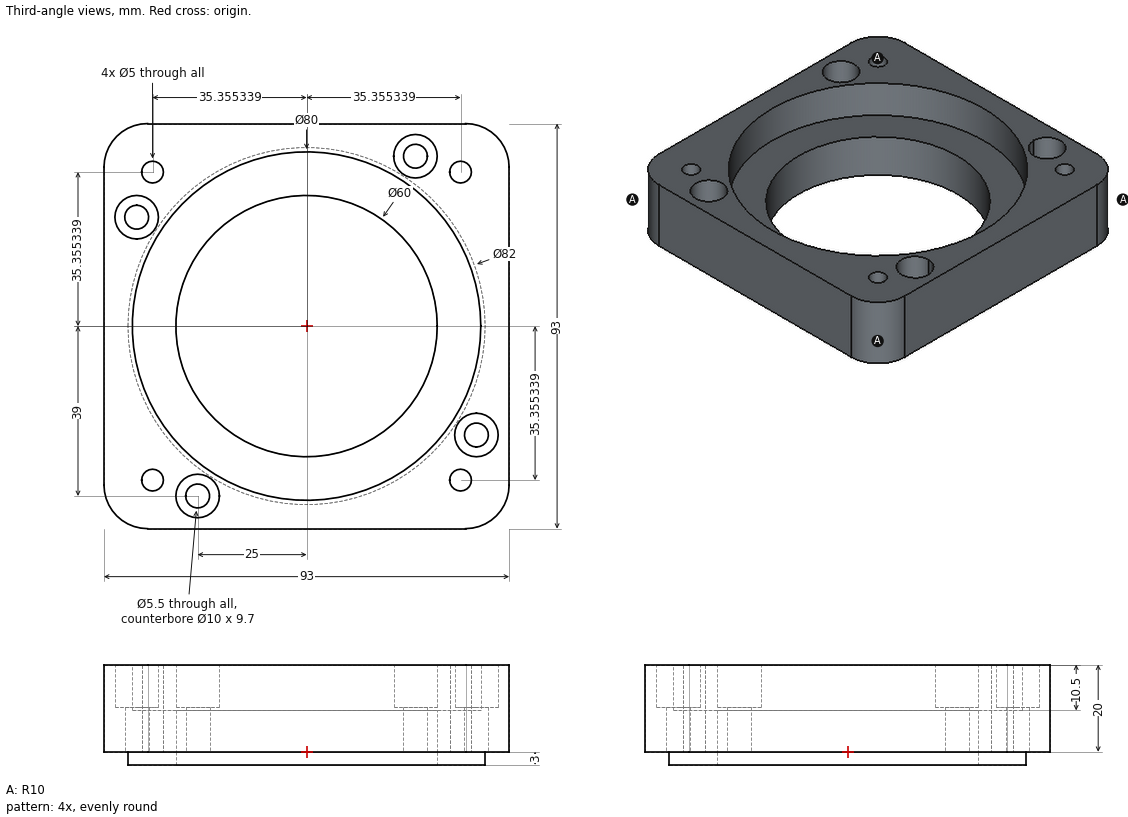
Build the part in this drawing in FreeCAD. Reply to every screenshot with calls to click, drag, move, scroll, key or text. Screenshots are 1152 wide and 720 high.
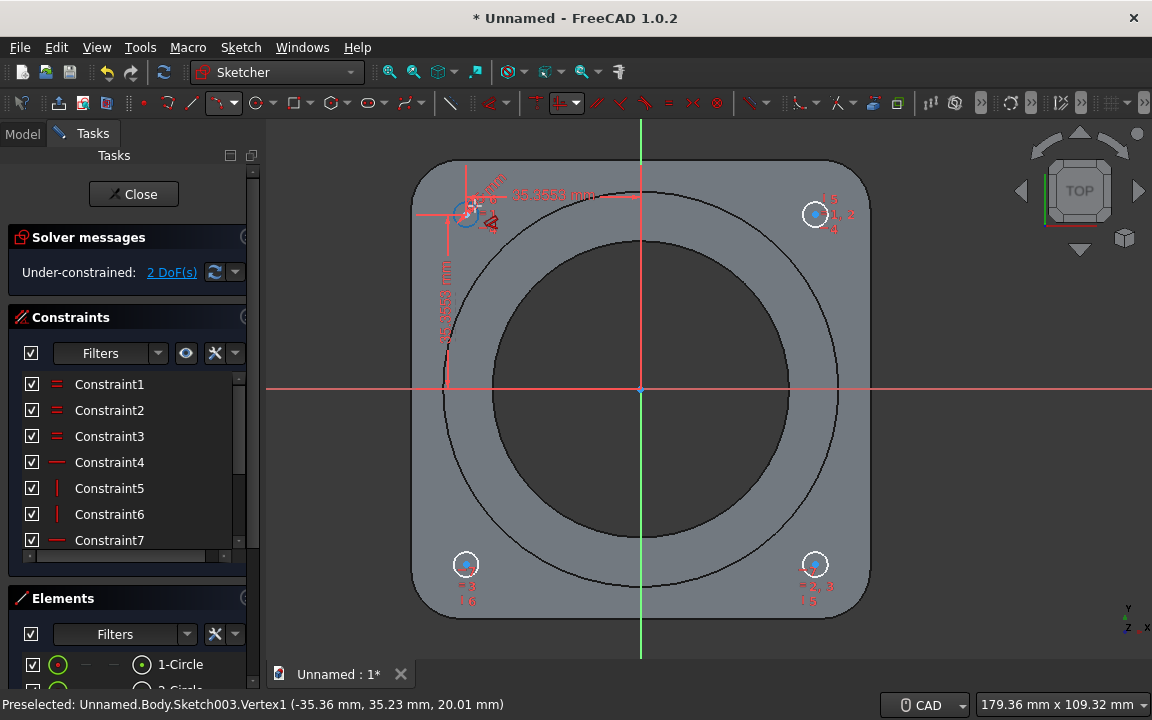
click(815, 215)
click(728, 181)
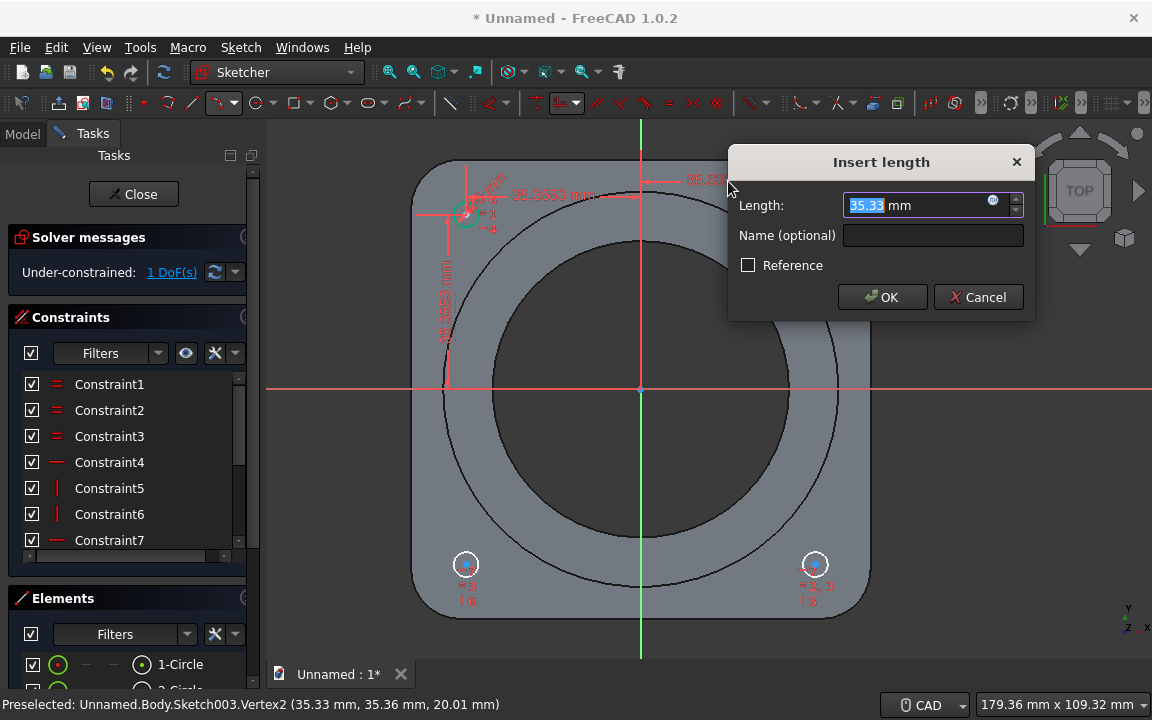
text(35.355339)
key(Return)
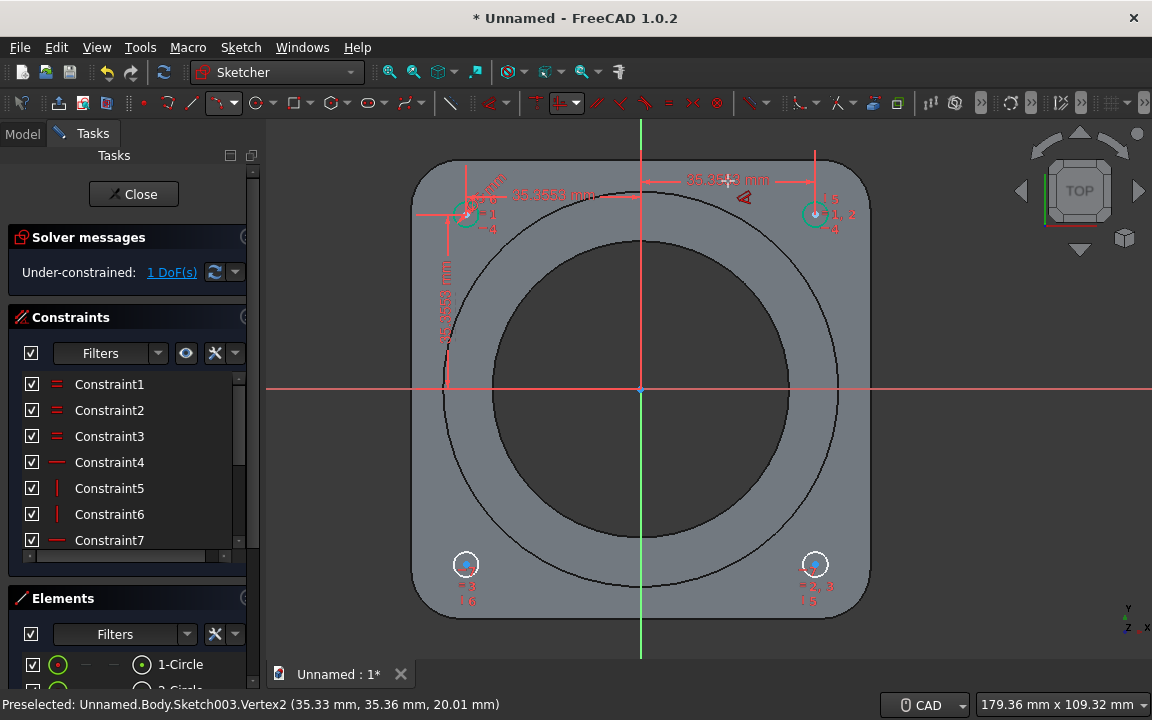
click(815, 565)
click(849, 477)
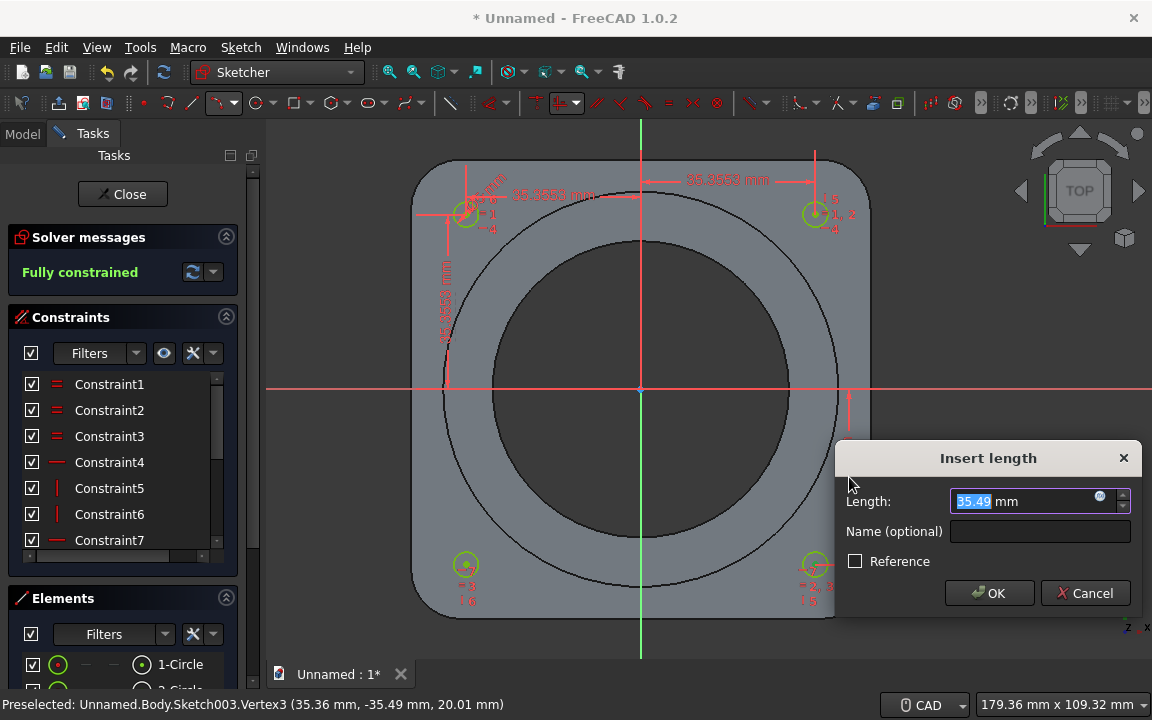
text(35.355339)
key(Return)
key(Escape)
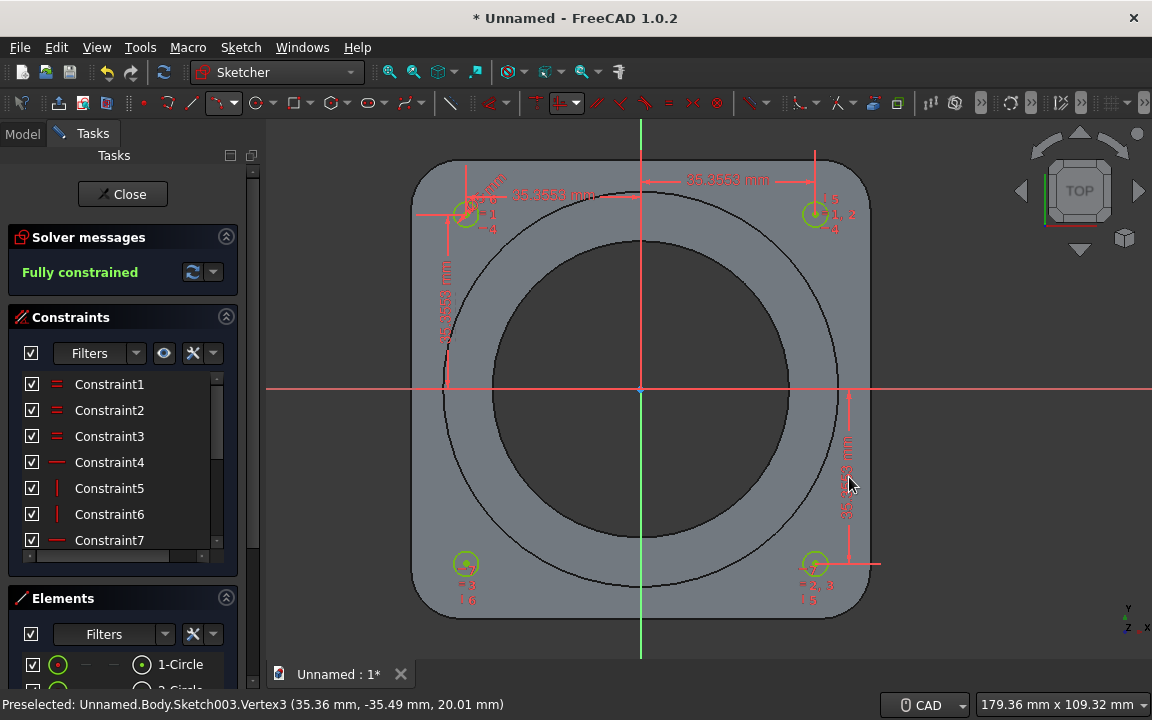
click(123, 194)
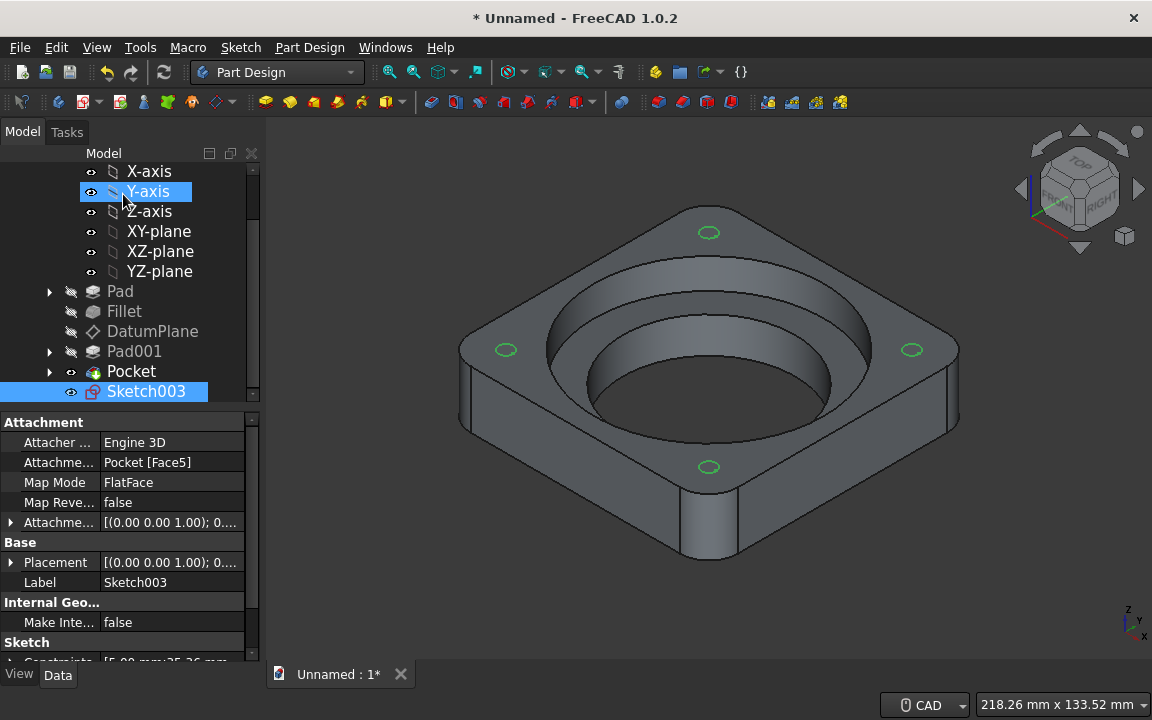
click(456, 102)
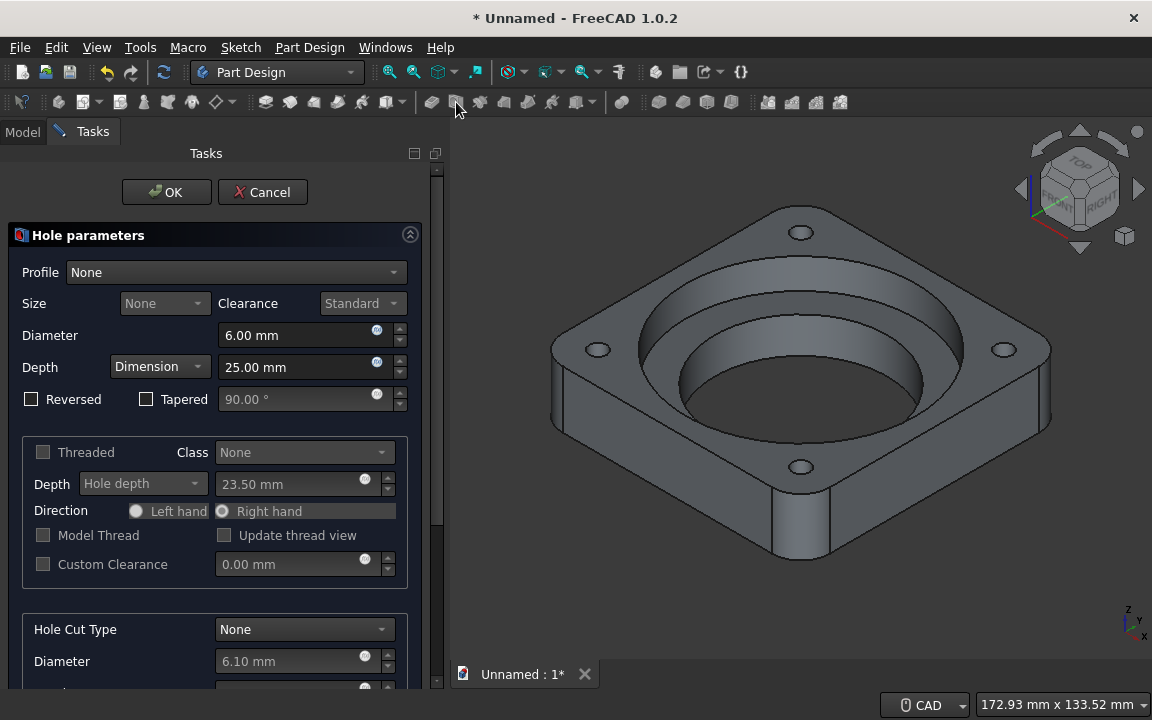
triple_click(305, 335)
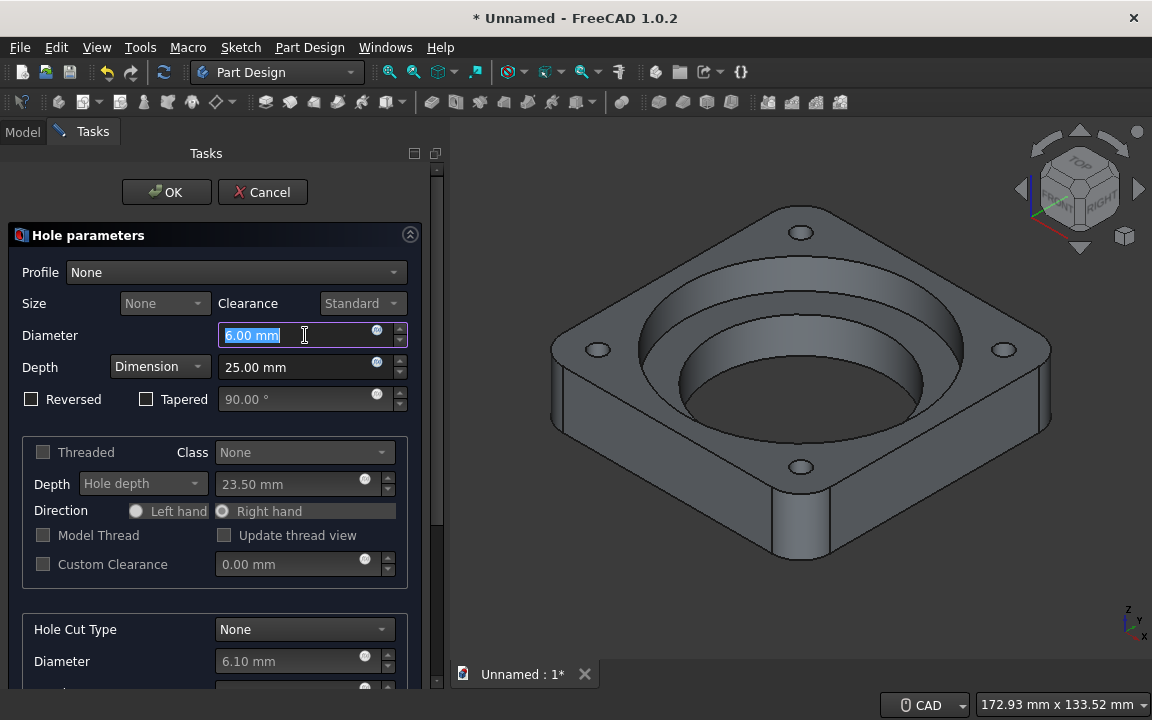
text(5)
key(Tab)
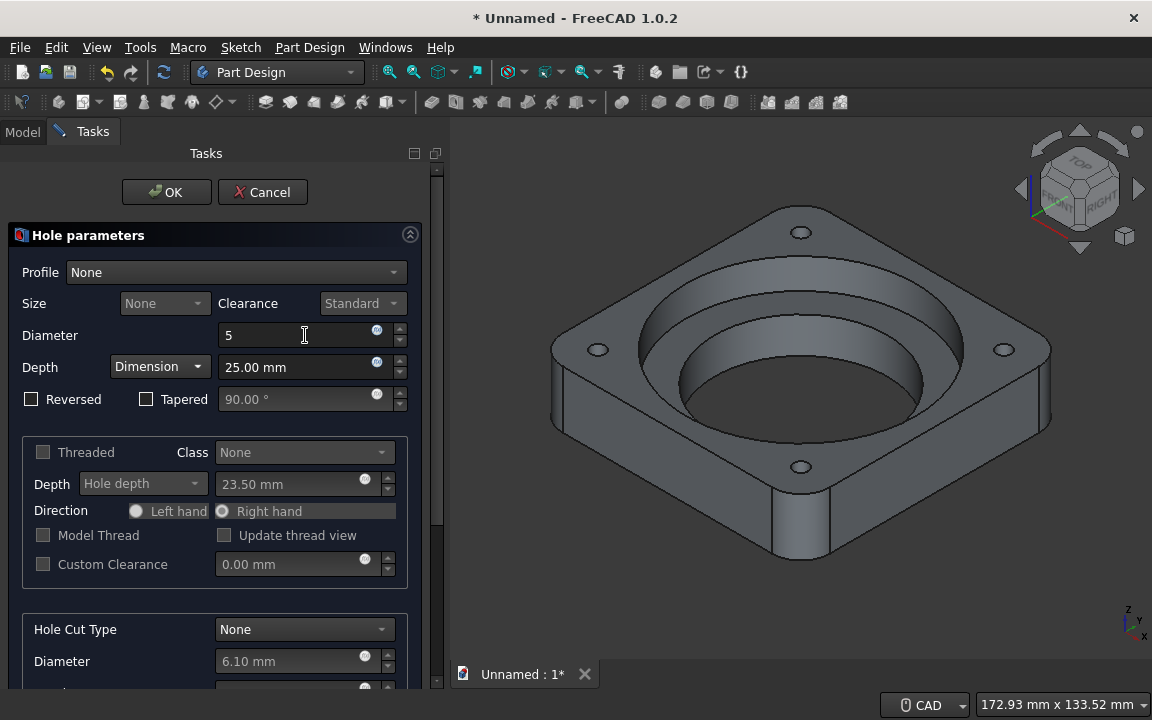
click(161, 366)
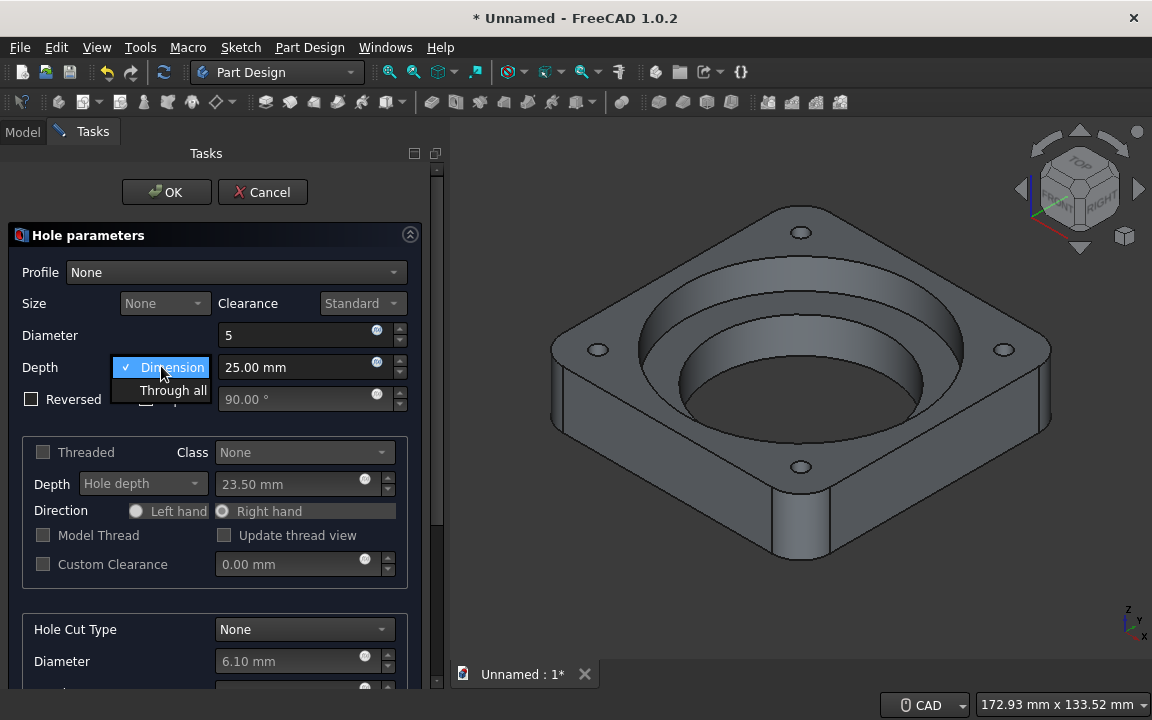
click(160, 390)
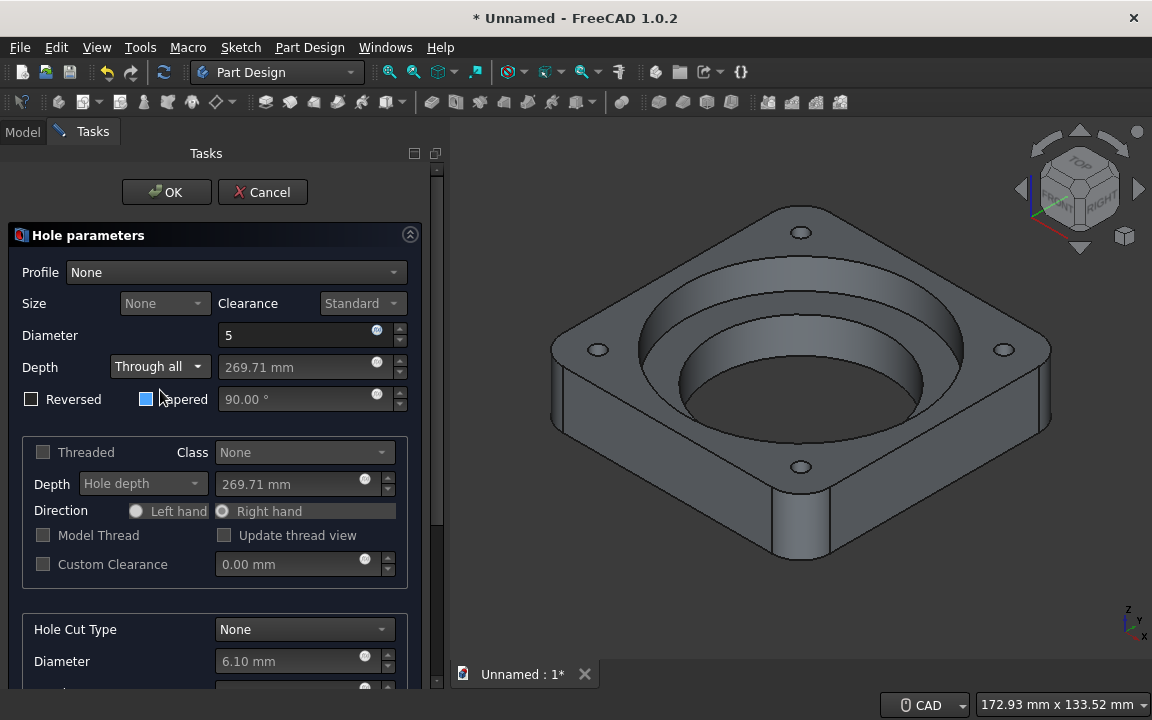
click(167, 192)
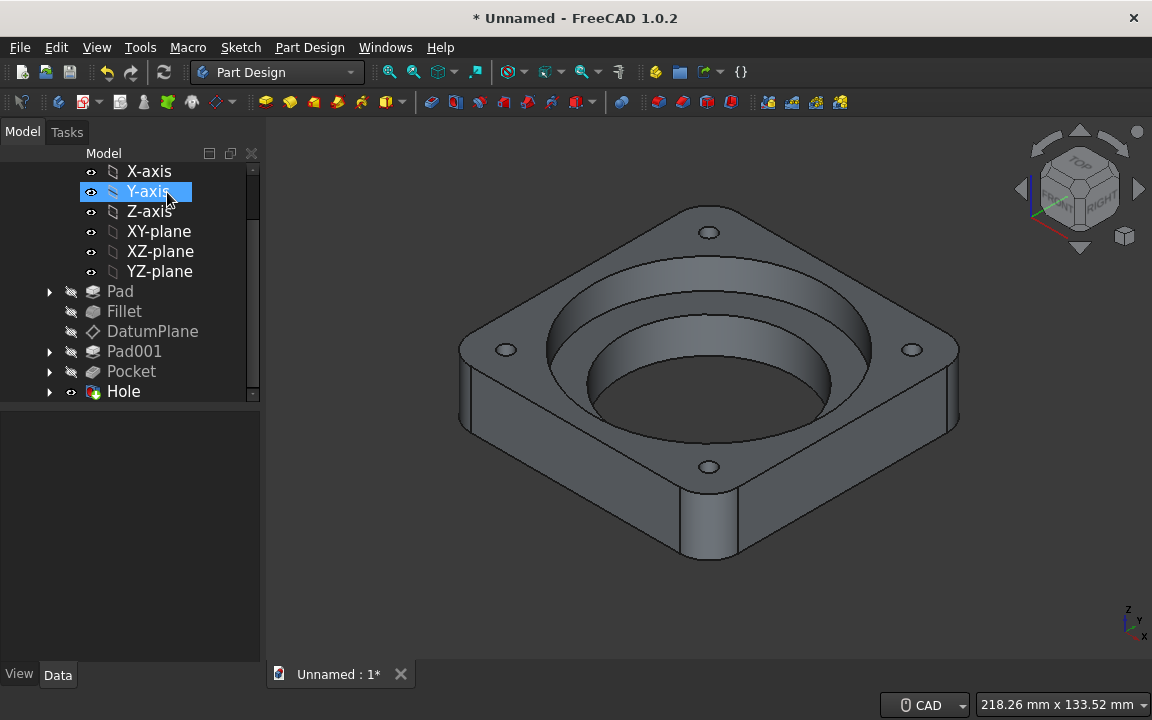
click(671, 459)